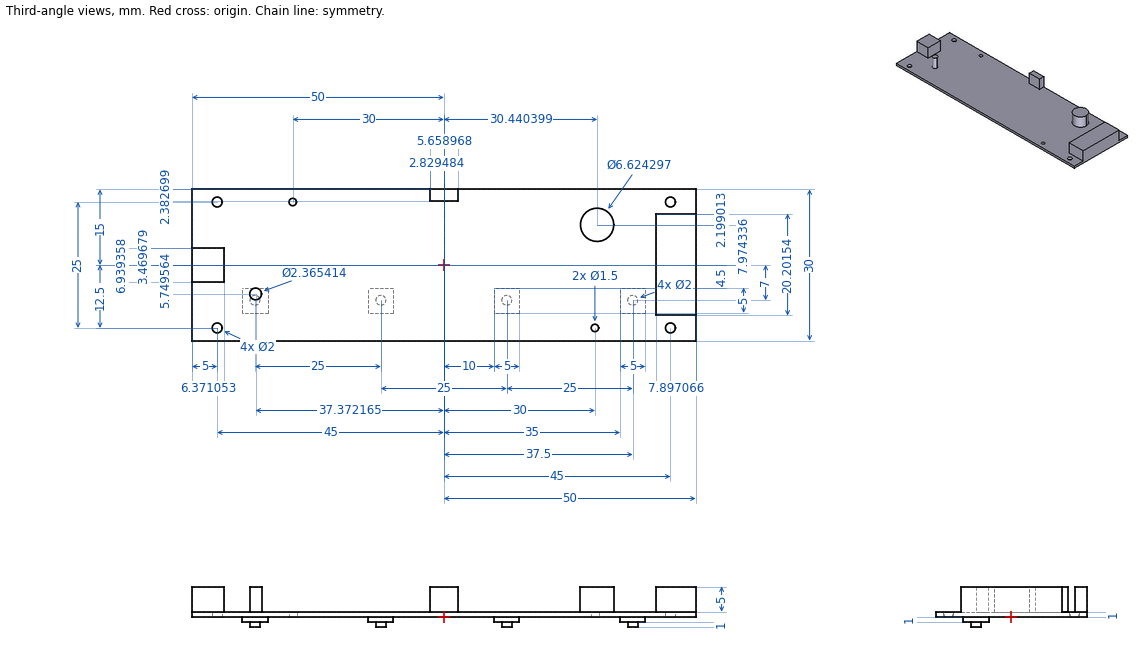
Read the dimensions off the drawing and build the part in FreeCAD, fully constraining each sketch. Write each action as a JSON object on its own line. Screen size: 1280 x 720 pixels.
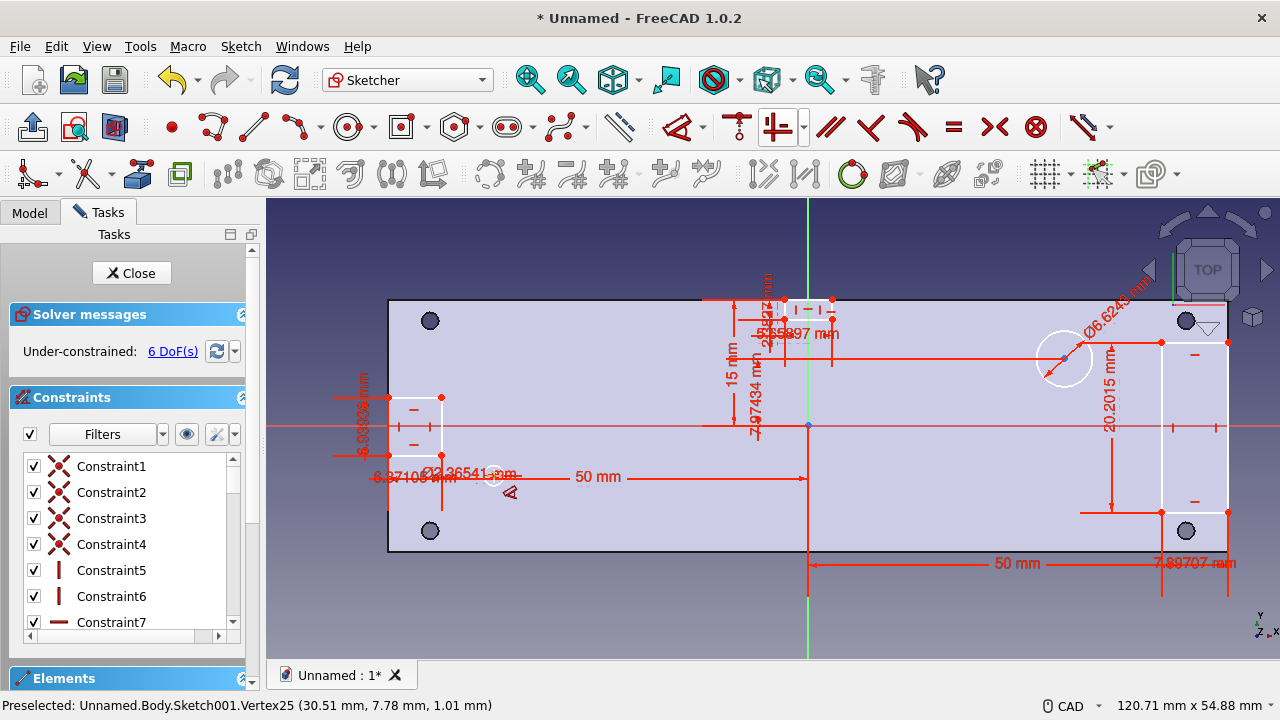
{"action": "left_click", "coordinate": [494, 476]}
{"action": "left_click", "coordinate": [460, 451]}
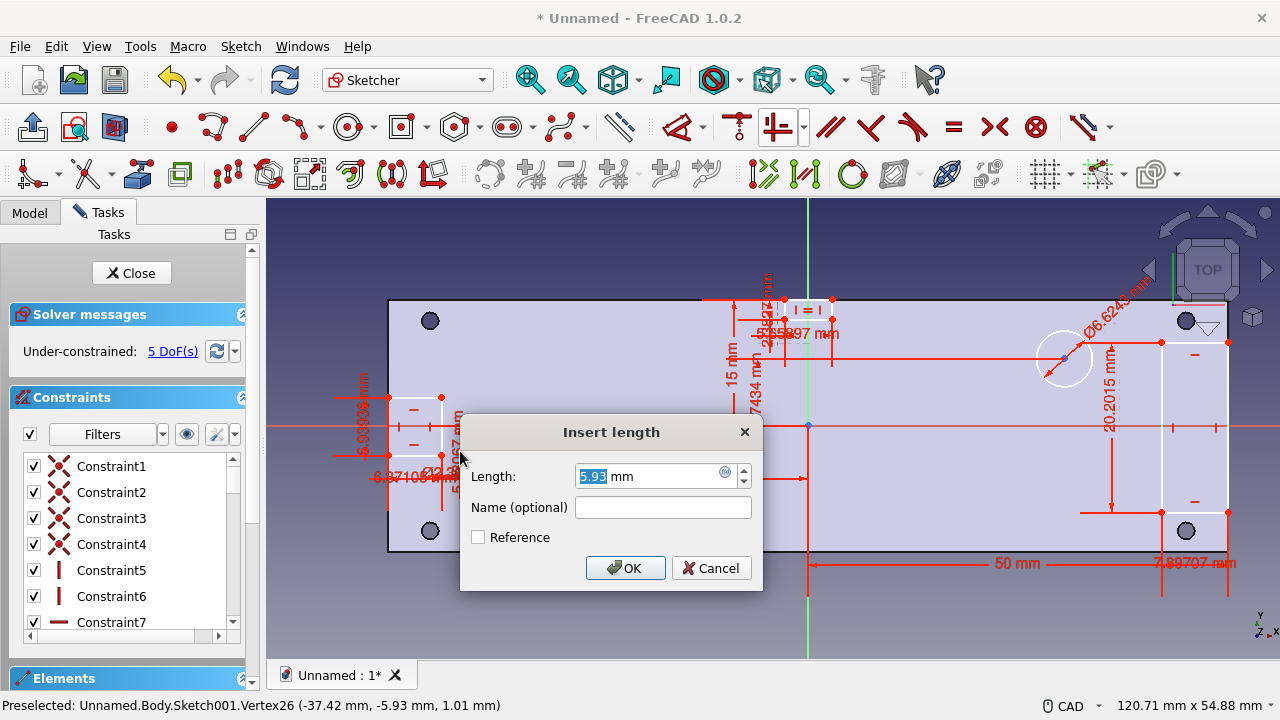
{"action": "type", "text": "5.749564"}
{"action": "key", "text": "Return"}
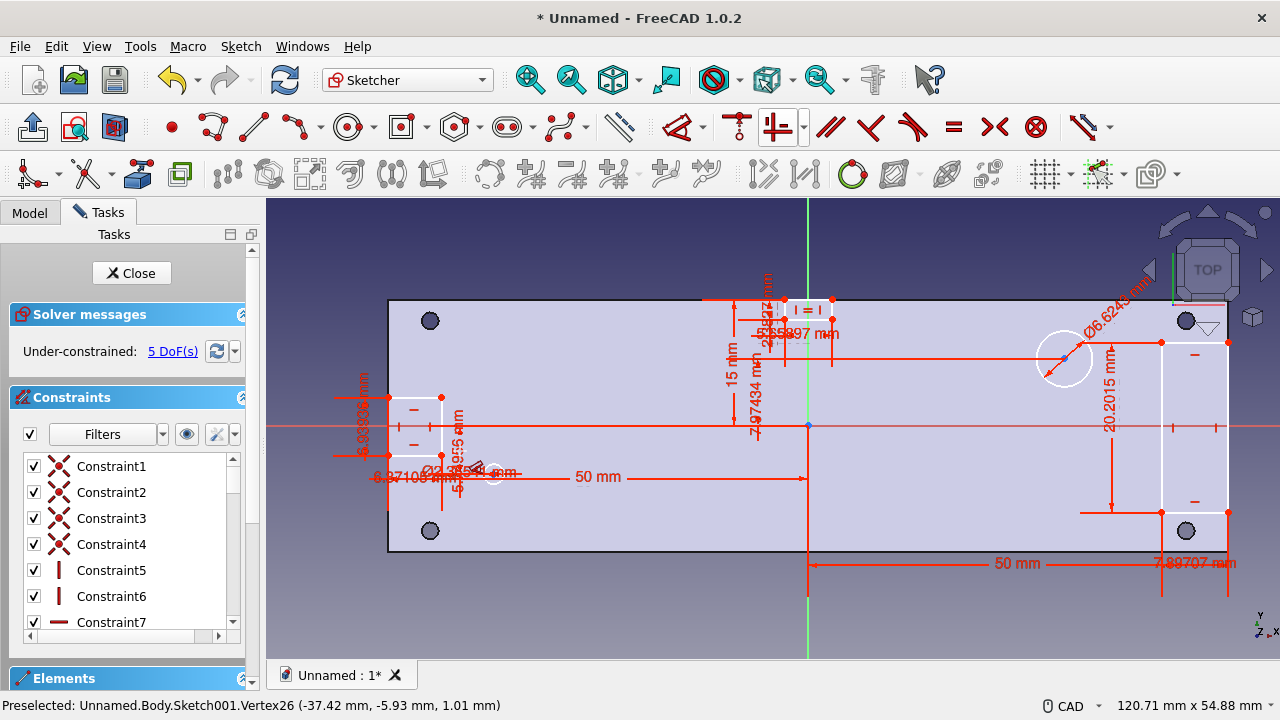
{"action": "scroll", "coordinate": [785, 300], "scroll_direction": "up", "scroll_amount": 3}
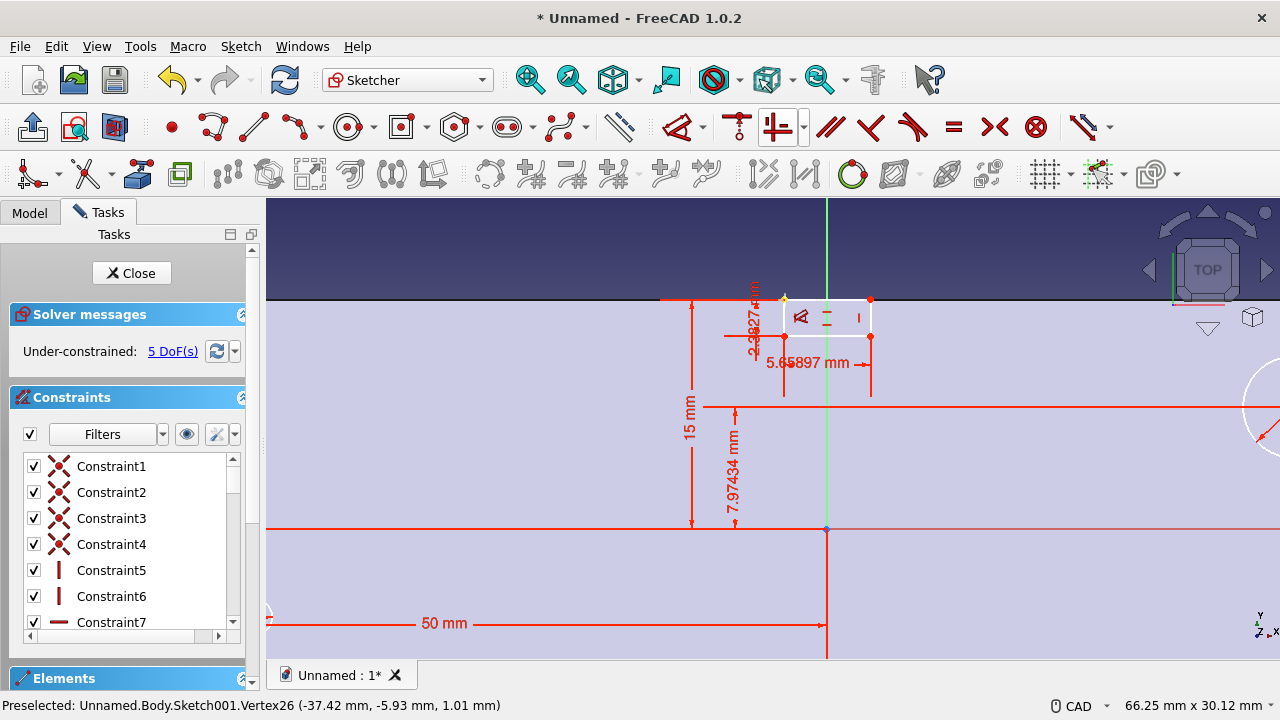
{"action": "left_click", "coordinate": [784, 300]}
{"action": "left_click", "coordinate": [806, 266]}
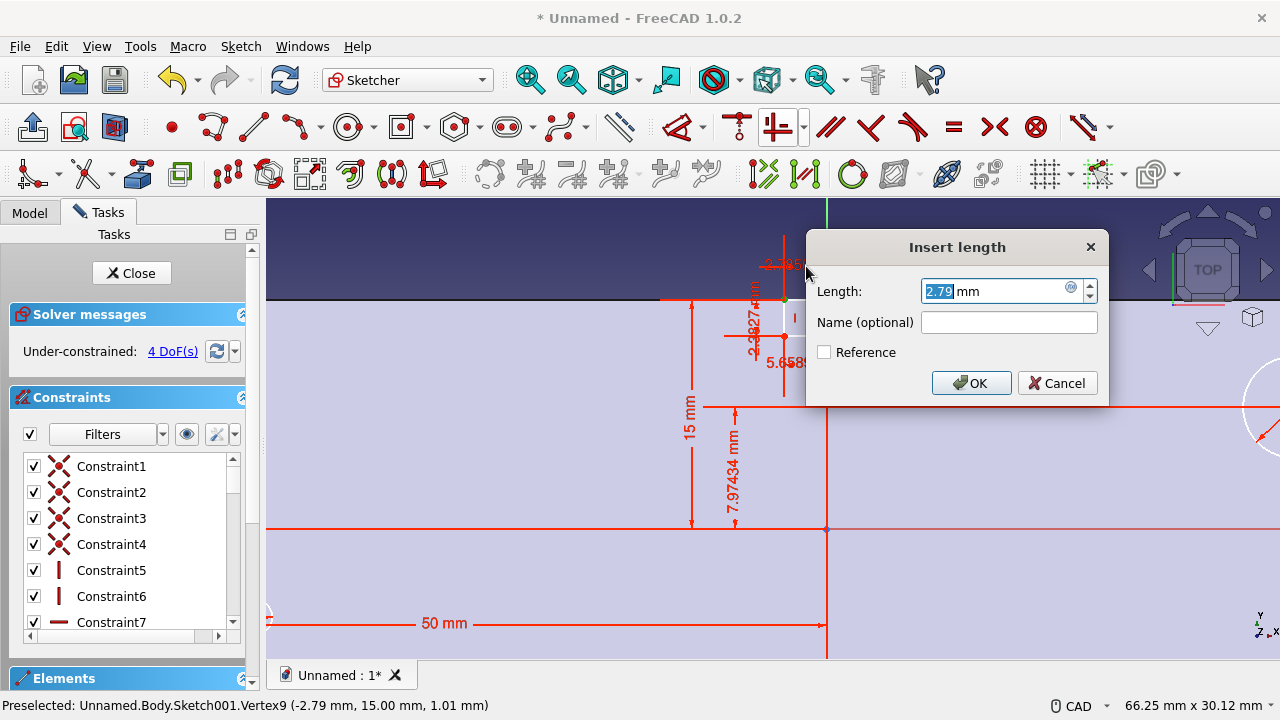
{"action": "type", "text": "2.829484"}
{"action": "key", "text": "Return"}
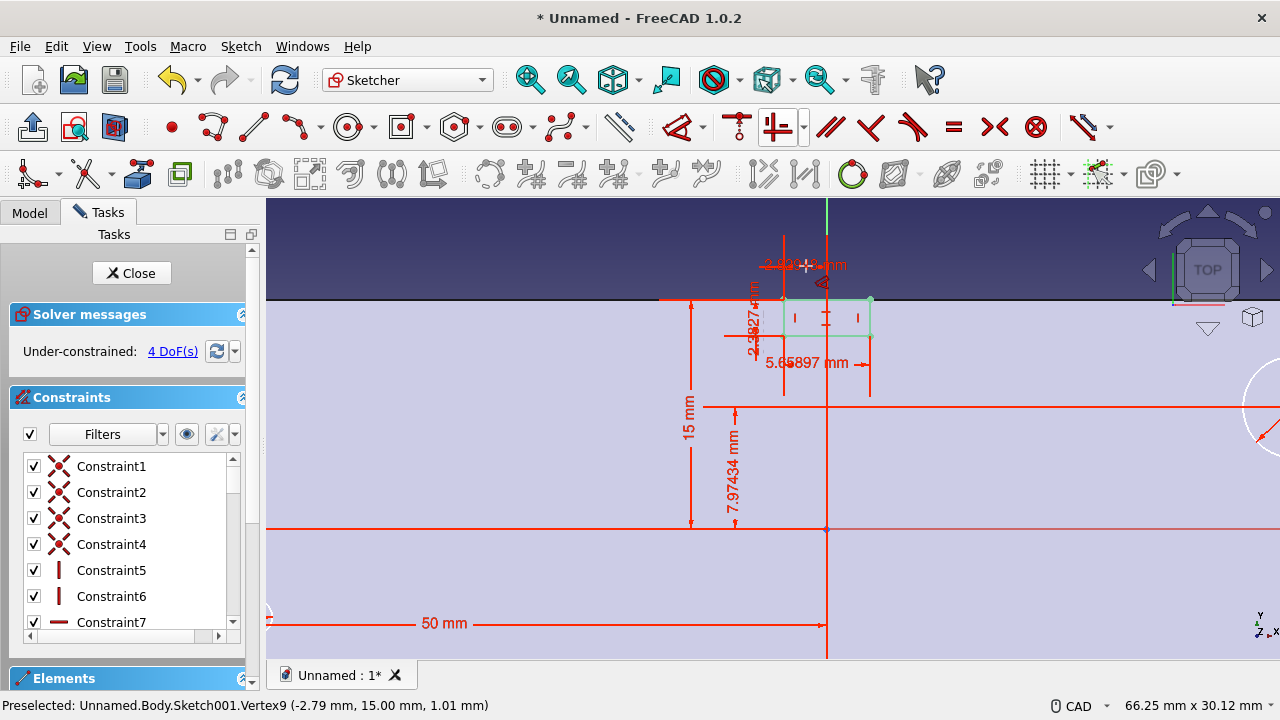
{"action": "scroll", "coordinate": [633, 392], "scroll_direction": "down", "scroll_amount": 5}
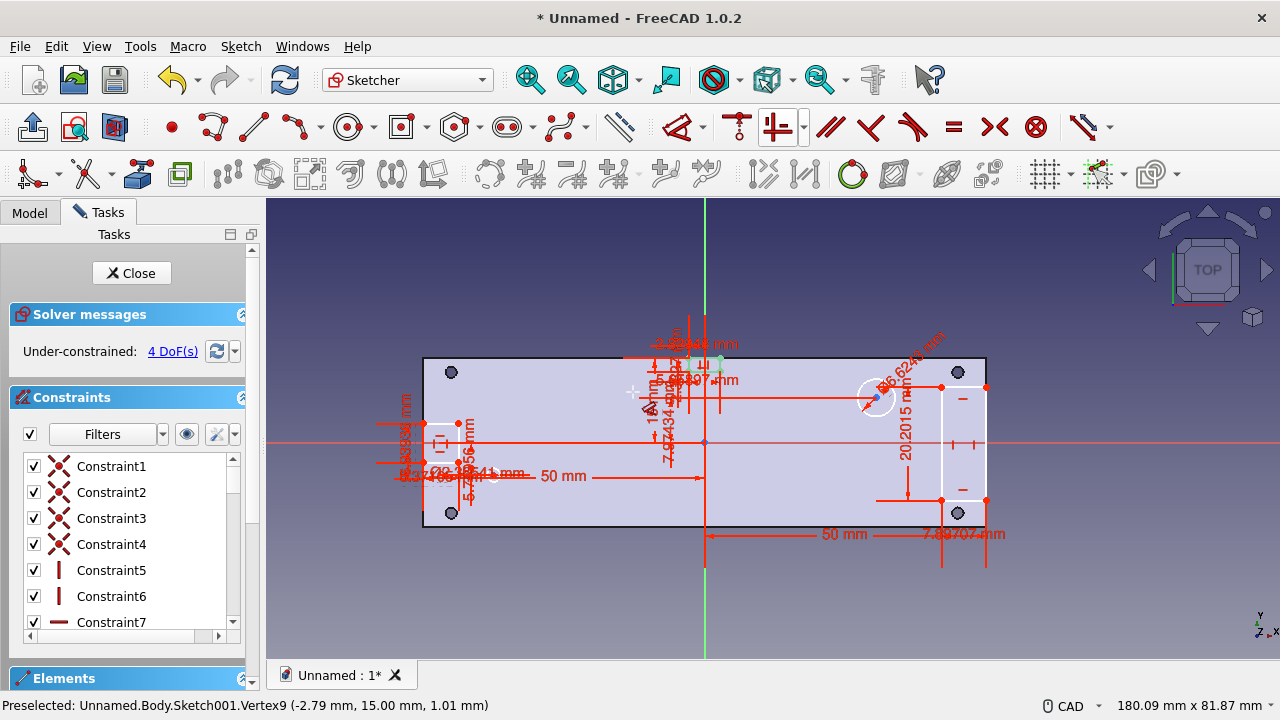
{"action": "scroll", "coordinate": [423, 424], "scroll_direction": "up", "scroll_amount": 4}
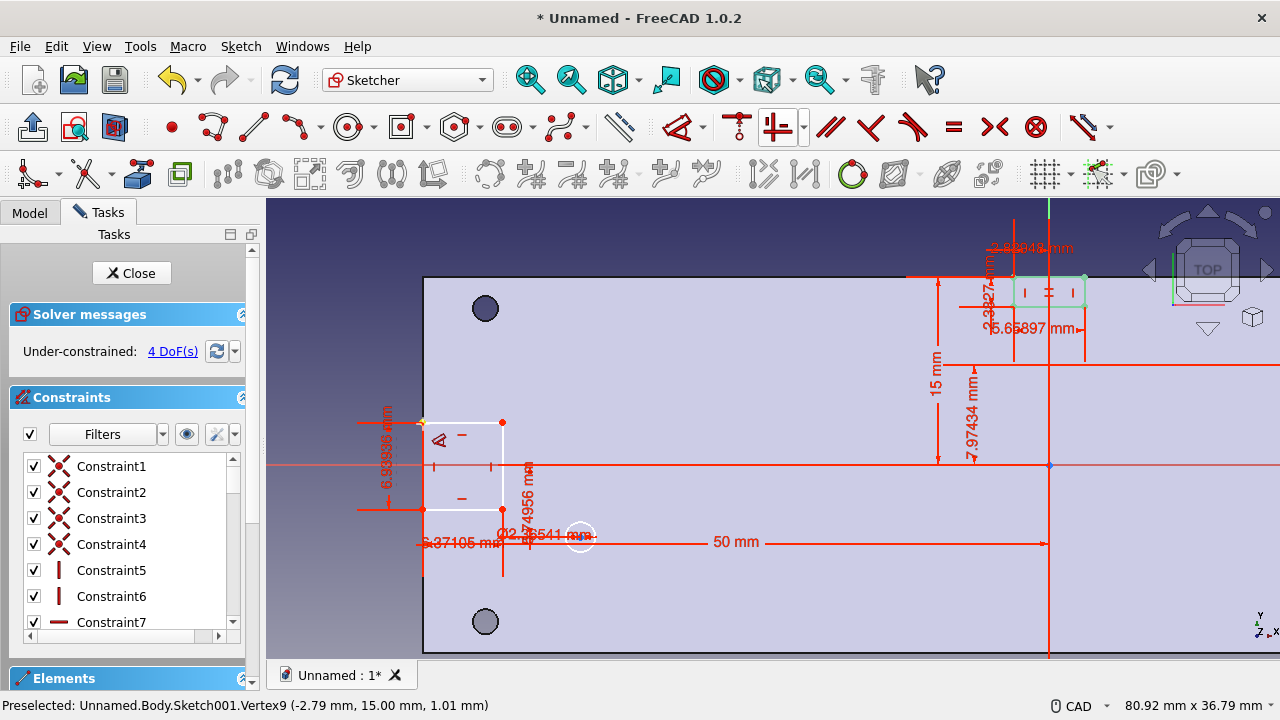
{"action": "left_click", "coordinate": [423, 423]}
{"action": "left_click", "coordinate": [1083, 444]}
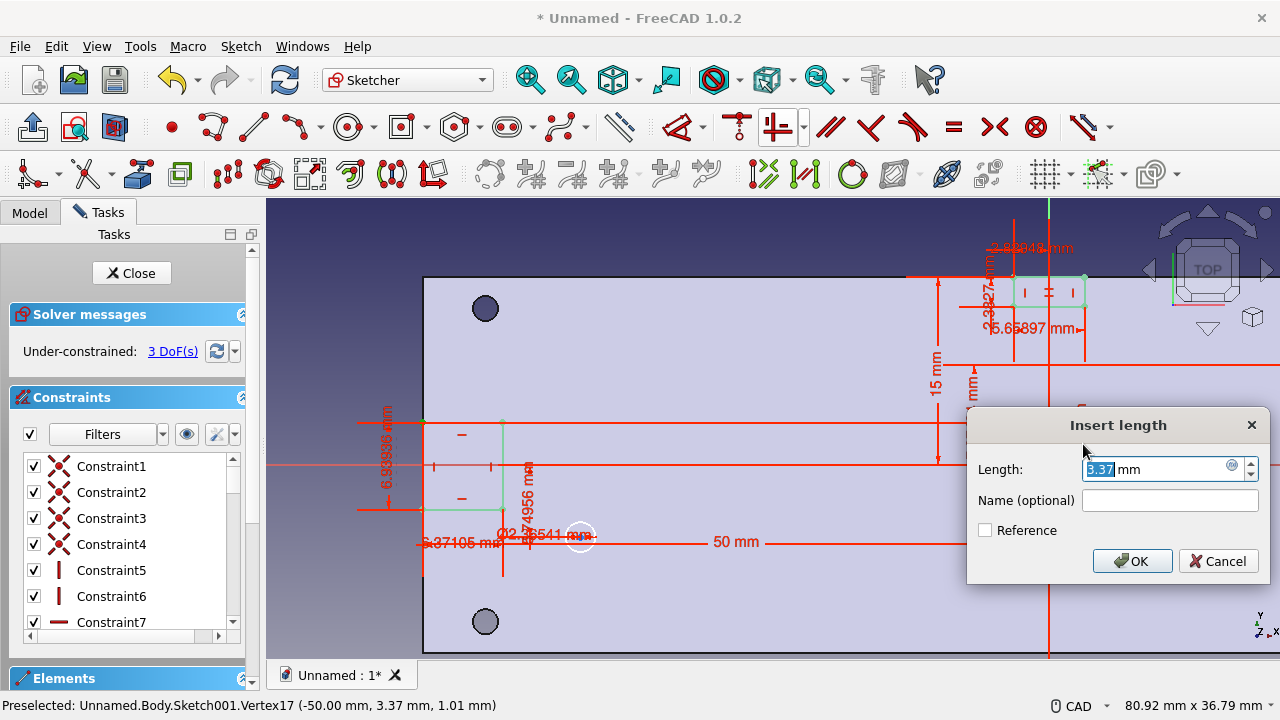
{"action": "type", "text": "3.469679"}
{"action": "key", "text": "Return"}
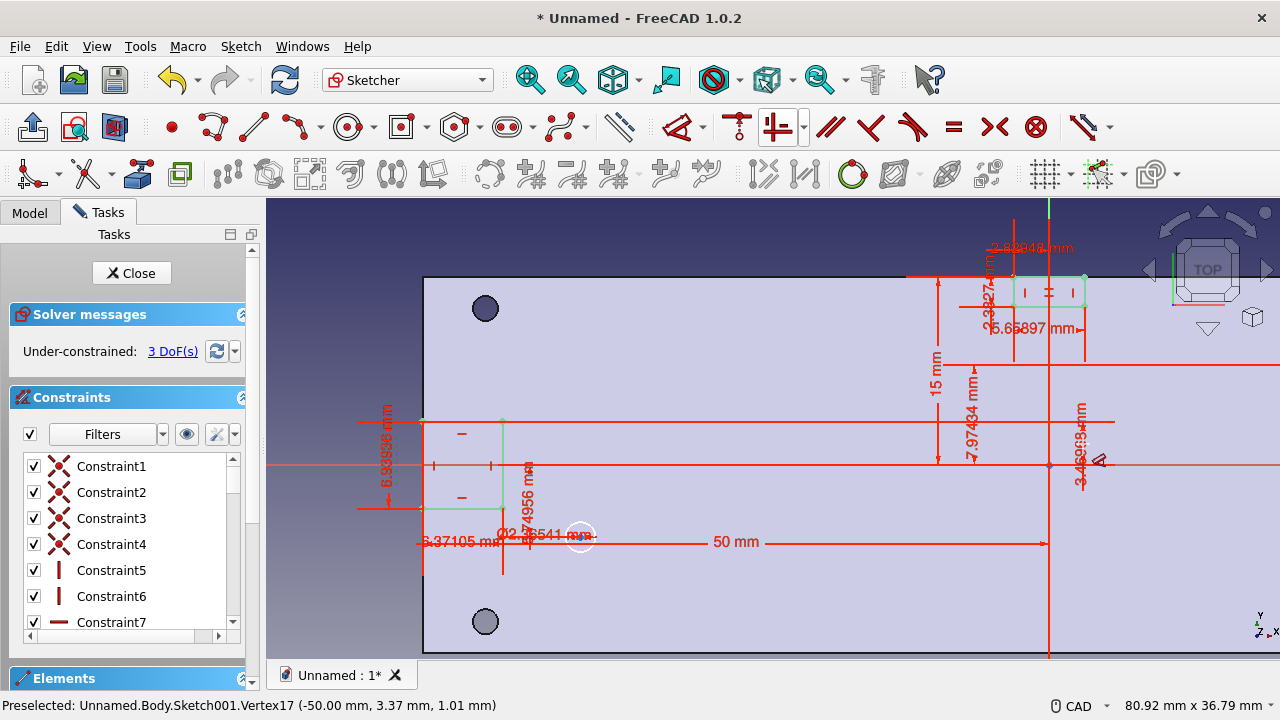
{"action": "scroll", "coordinate": [423, 424], "scroll_direction": "down", "scroll_amount": 4}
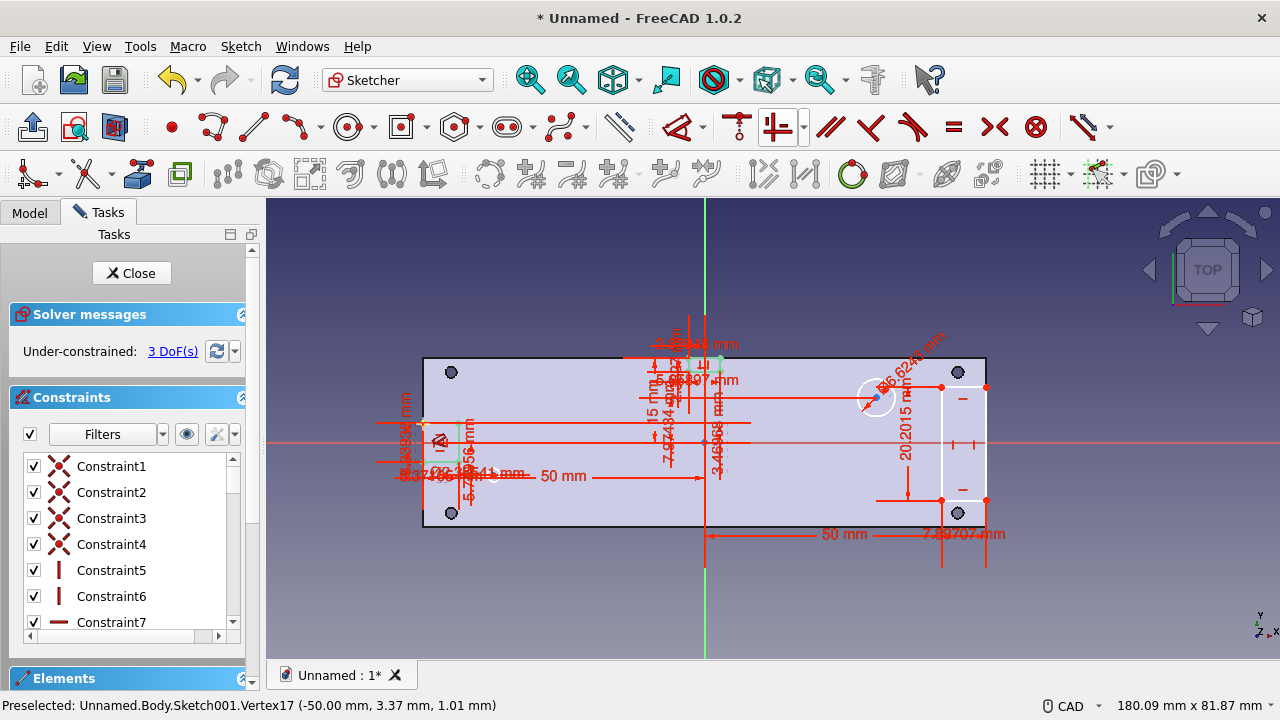
{"action": "left_click", "coordinate": [876, 398]}
{"action": "left_click", "coordinate": [790, 364]}